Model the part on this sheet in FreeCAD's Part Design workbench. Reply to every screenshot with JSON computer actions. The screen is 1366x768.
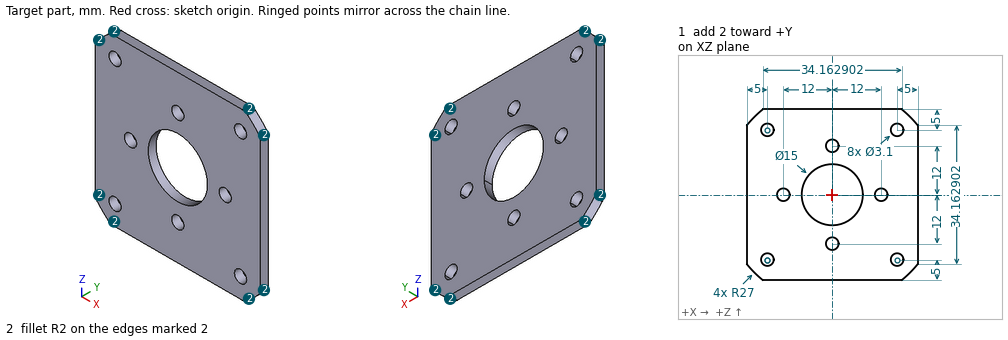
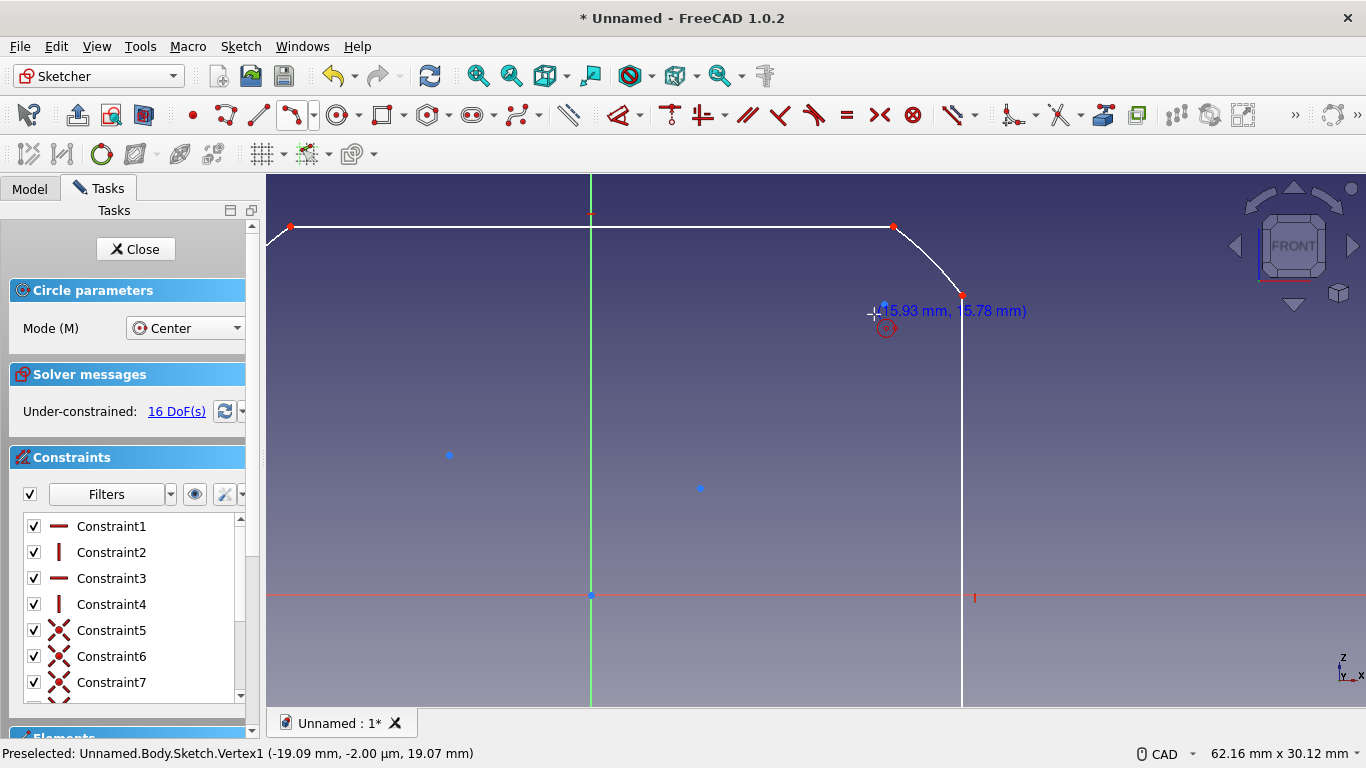
{"action": "left_click", "coordinate": [873, 314]}
{"action": "mouse_move", "coordinate": [892, 294]}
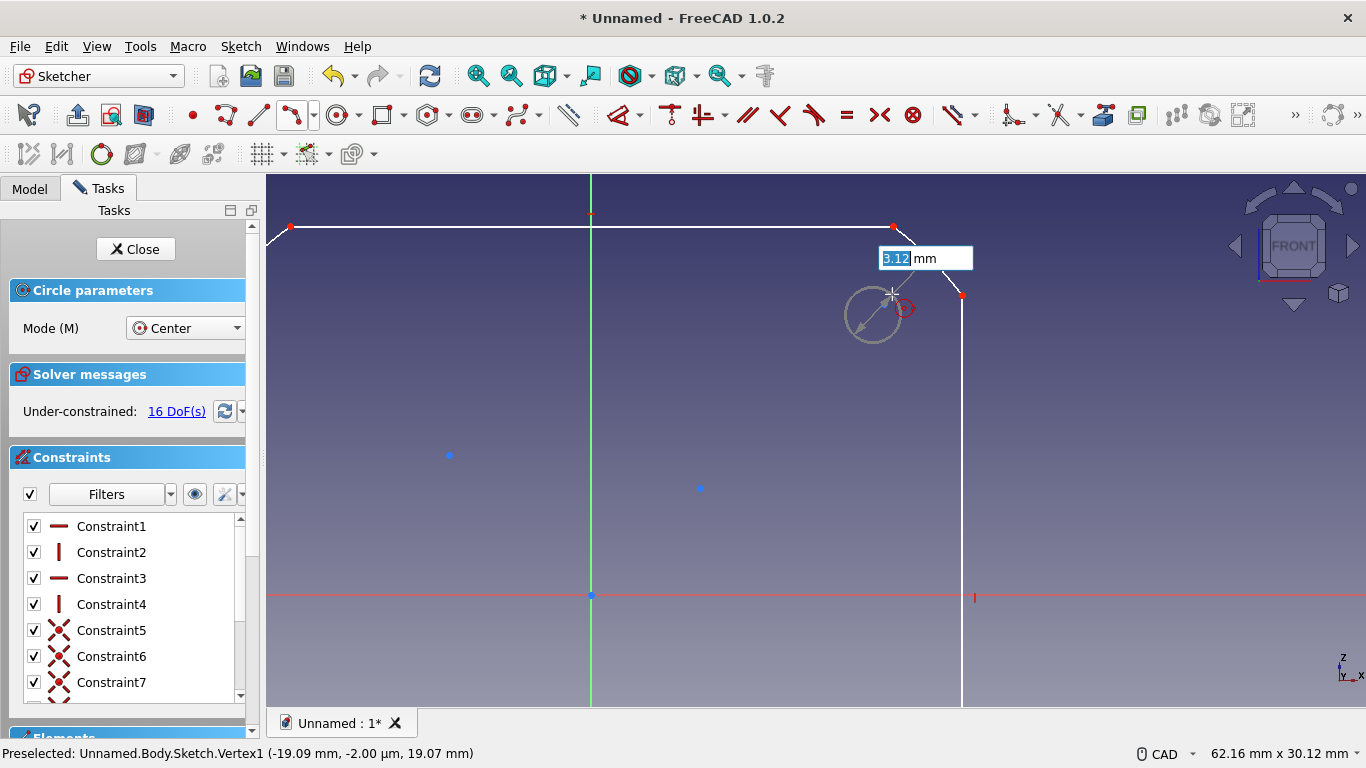
{"action": "type", "text": "3.1"}
{"action": "key", "text": "Return"}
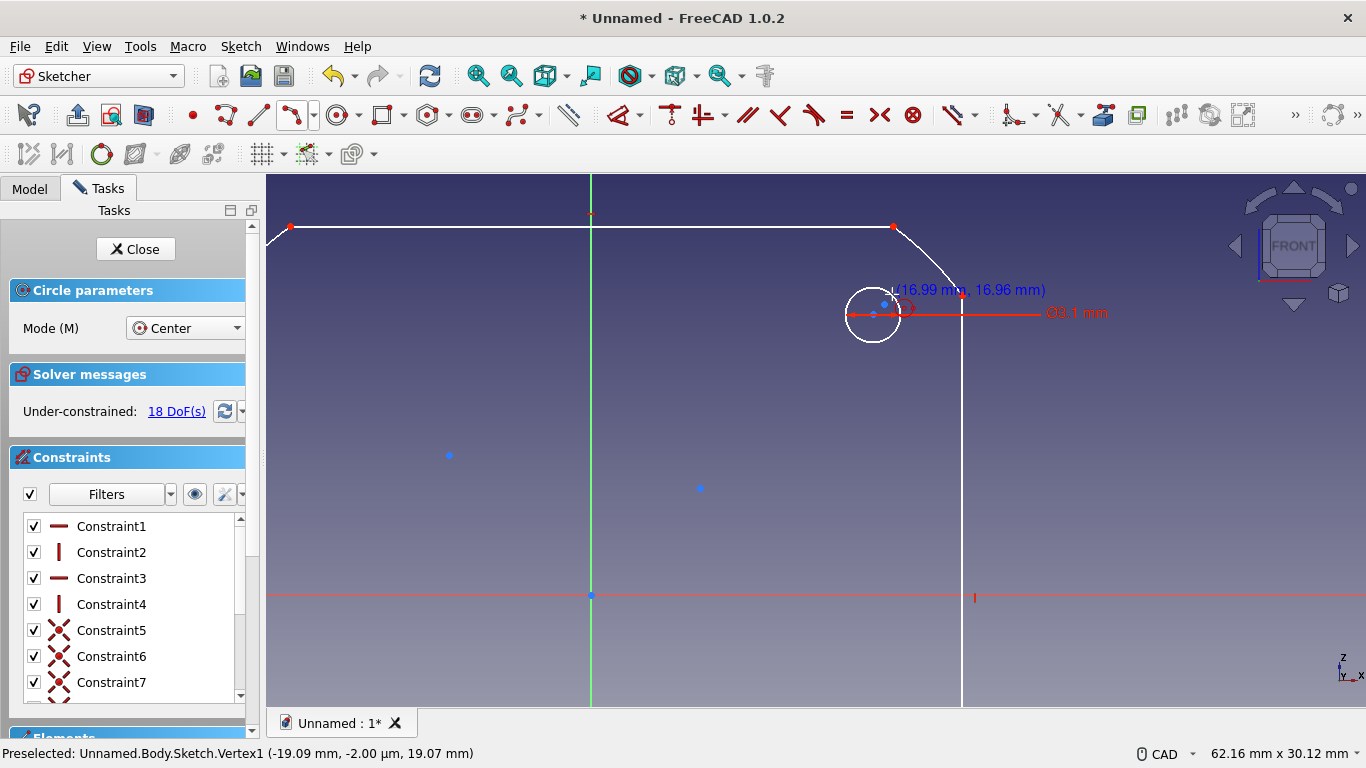
{"action": "left_click", "coordinate": [591, 383]}
{"action": "mouse_move", "coordinate": [611, 363]}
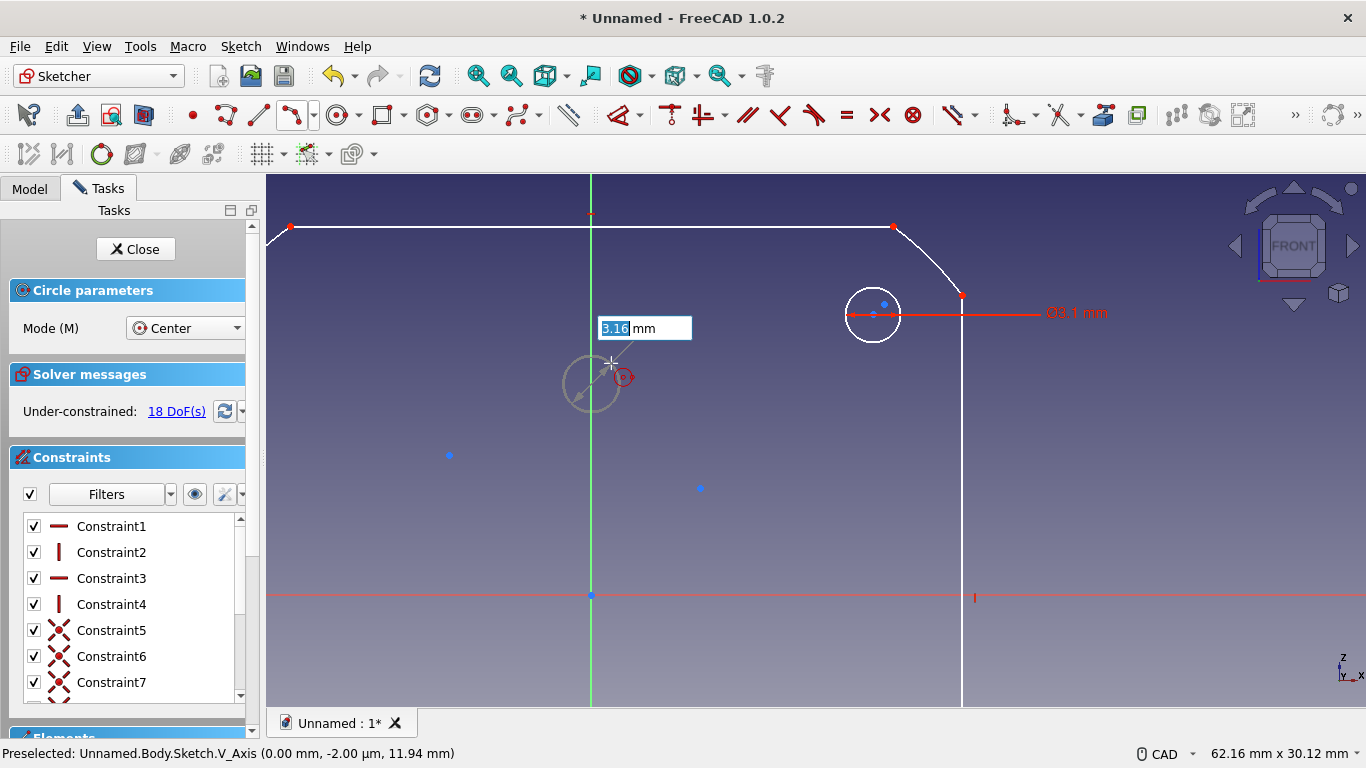
{"action": "type", "text": "3.1"}
{"action": "key", "text": "Return"}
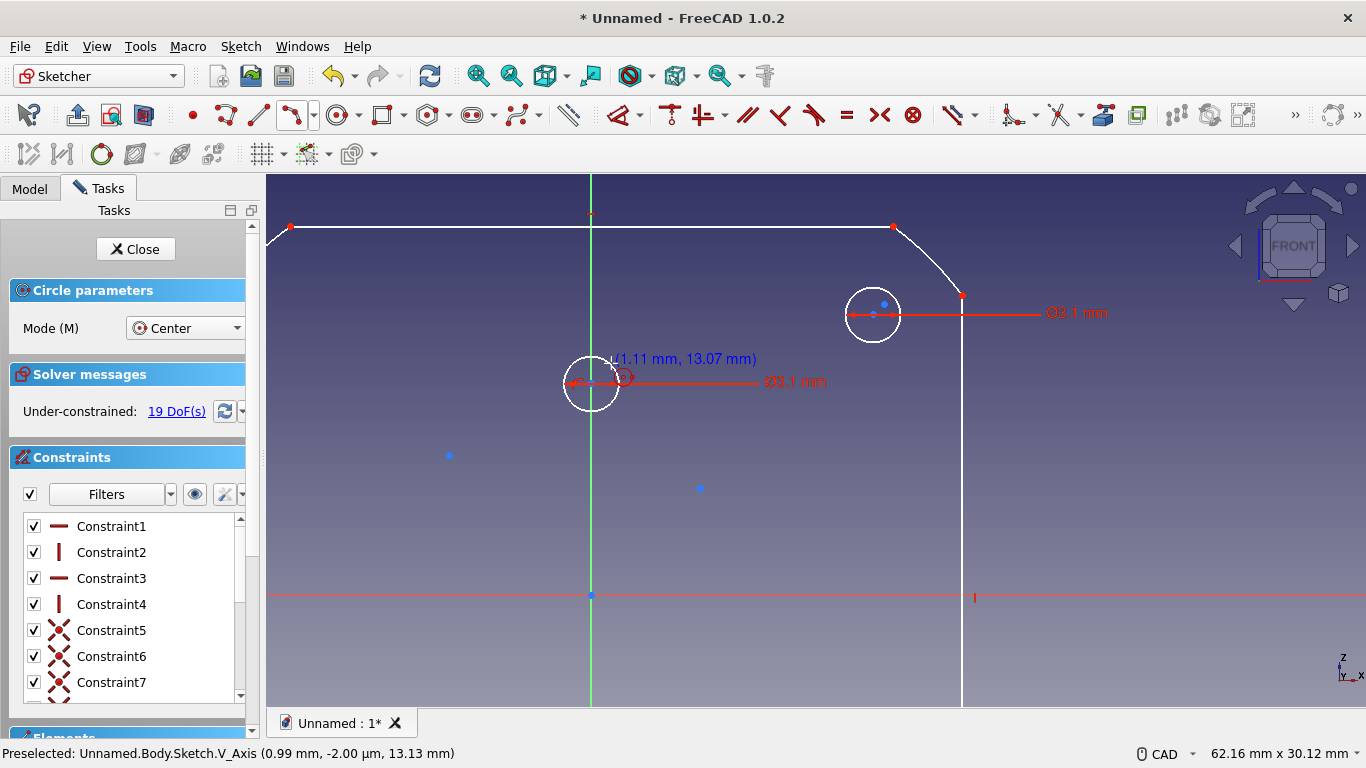
{"action": "left_click", "coordinate": [310, 314]}
{"action": "mouse_move", "coordinate": [329, 294]}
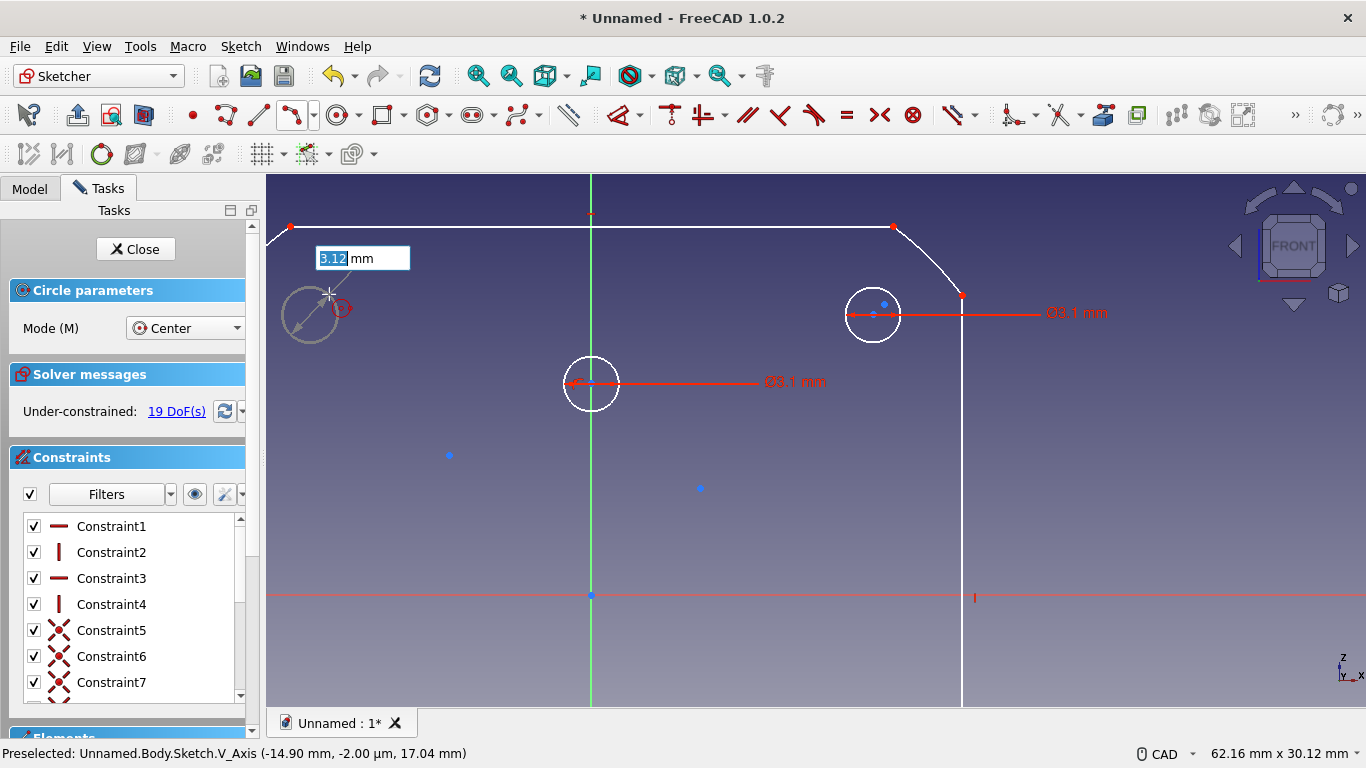
{"action": "type", "text": "3.1"}
{"action": "key", "text": "Return"}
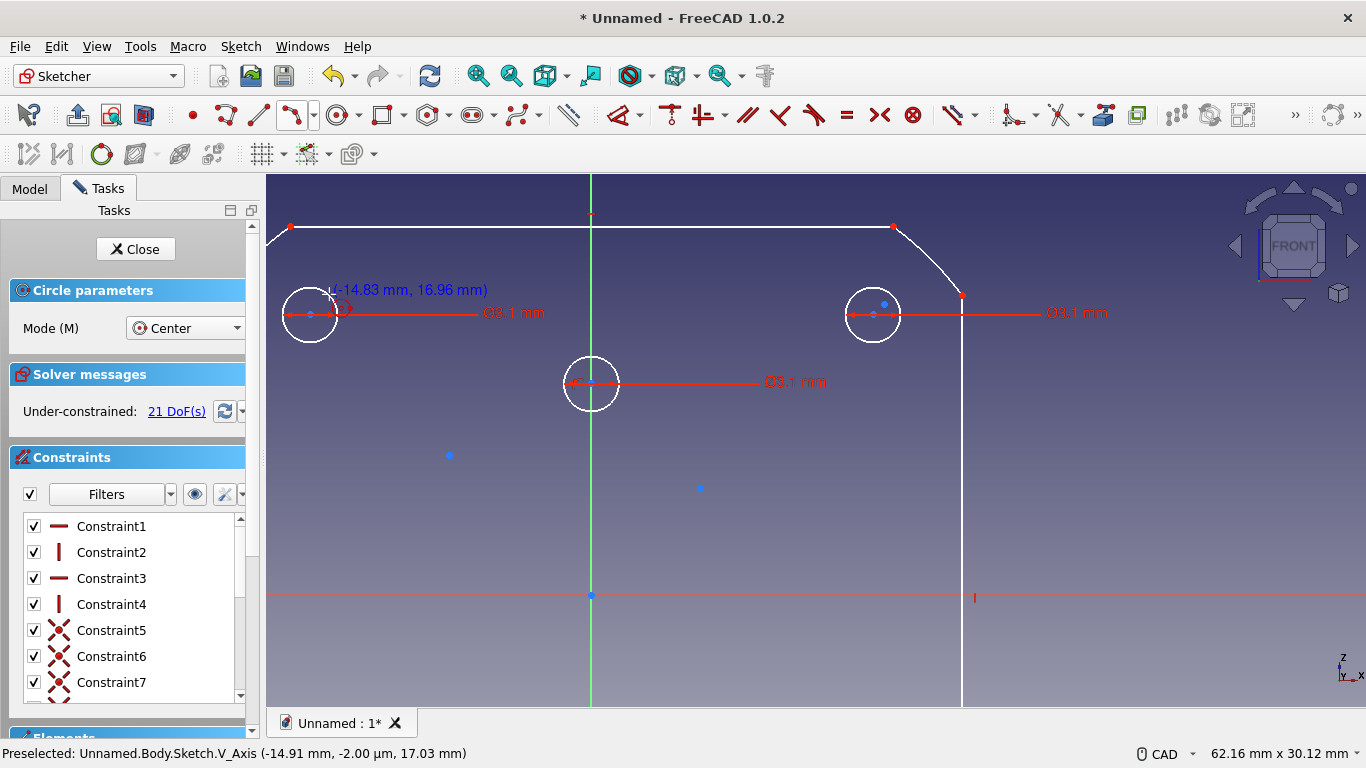
{"action": "left_click", "coordinate": [804, 595]}
{"action": "mouse_move", "coordinate": [823, 576]}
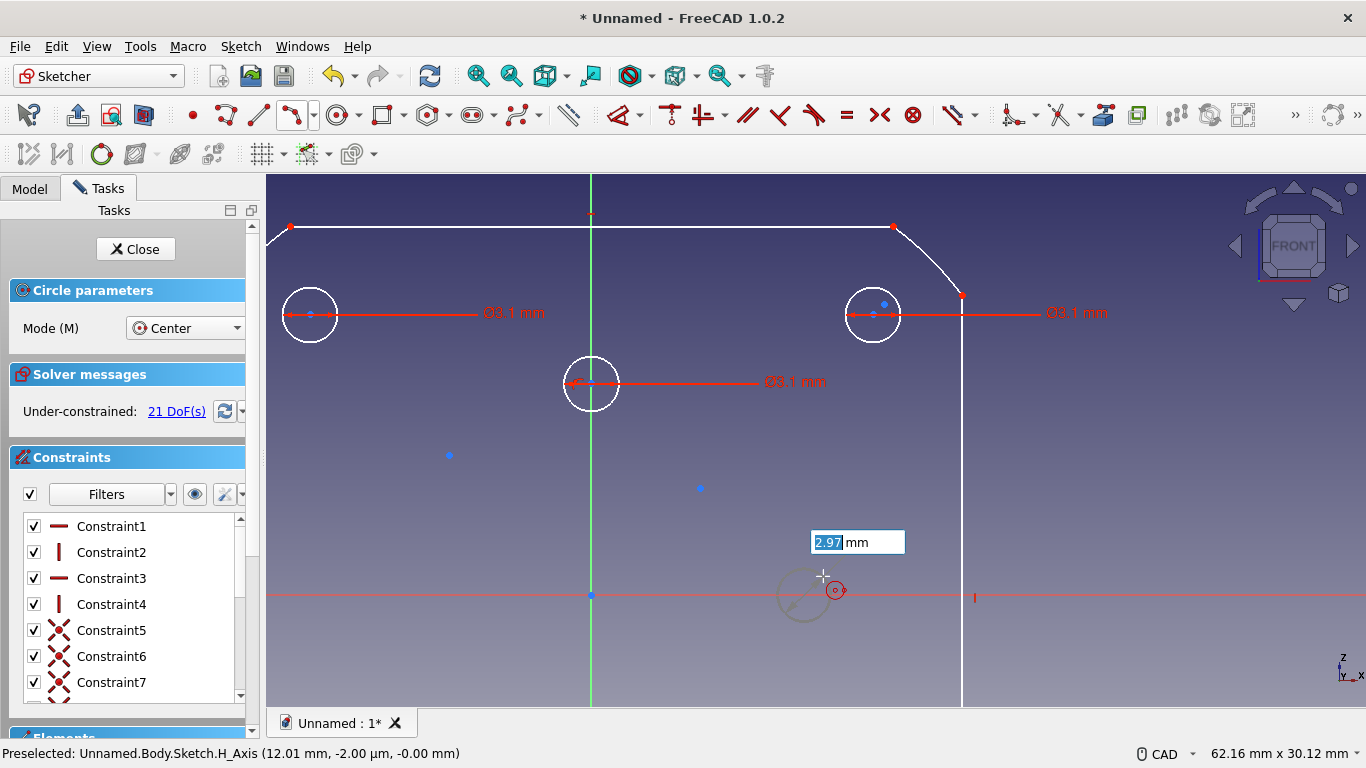
{"action": "type", "text": "3.1"}
{"action": "key", "text": "Return"}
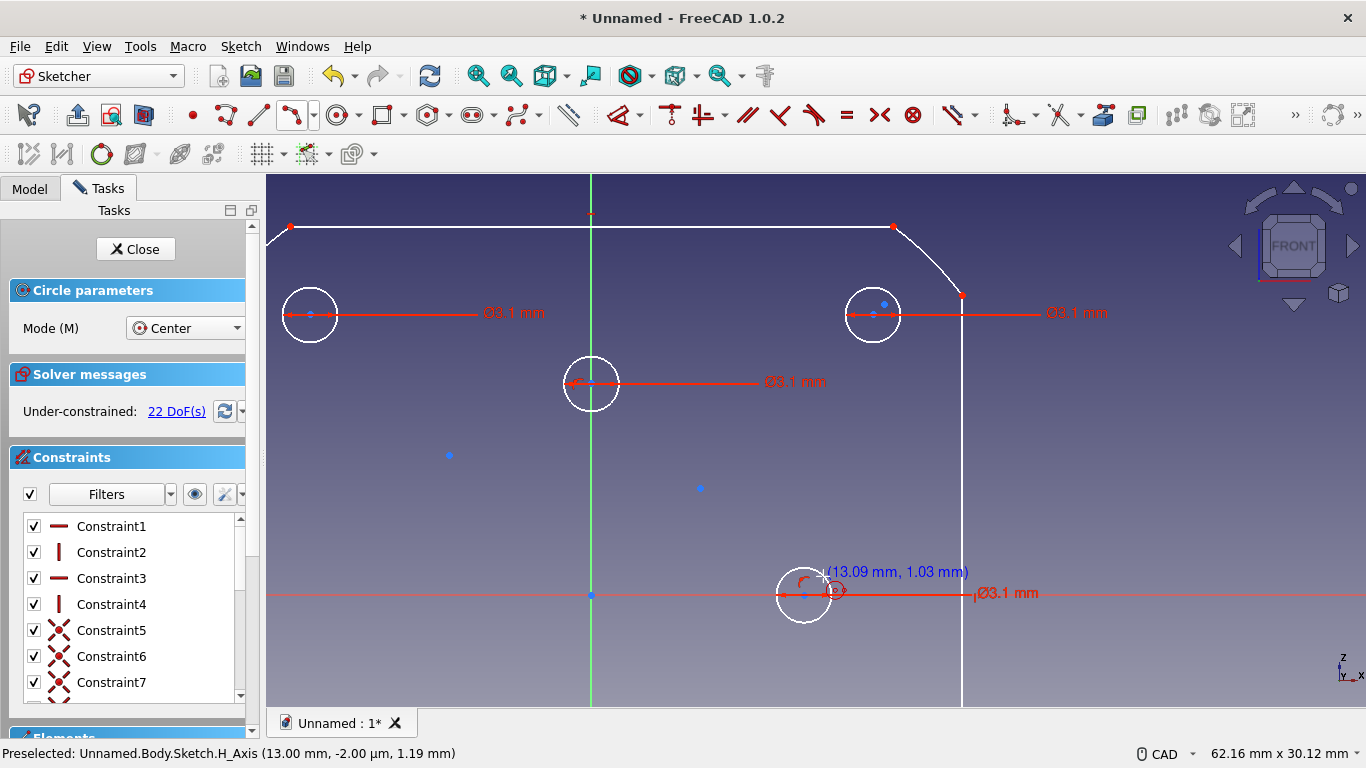
{"action": "scroll", "coordinate": [875, 314], "scroll_direction": "down", "scroll_amount": 4}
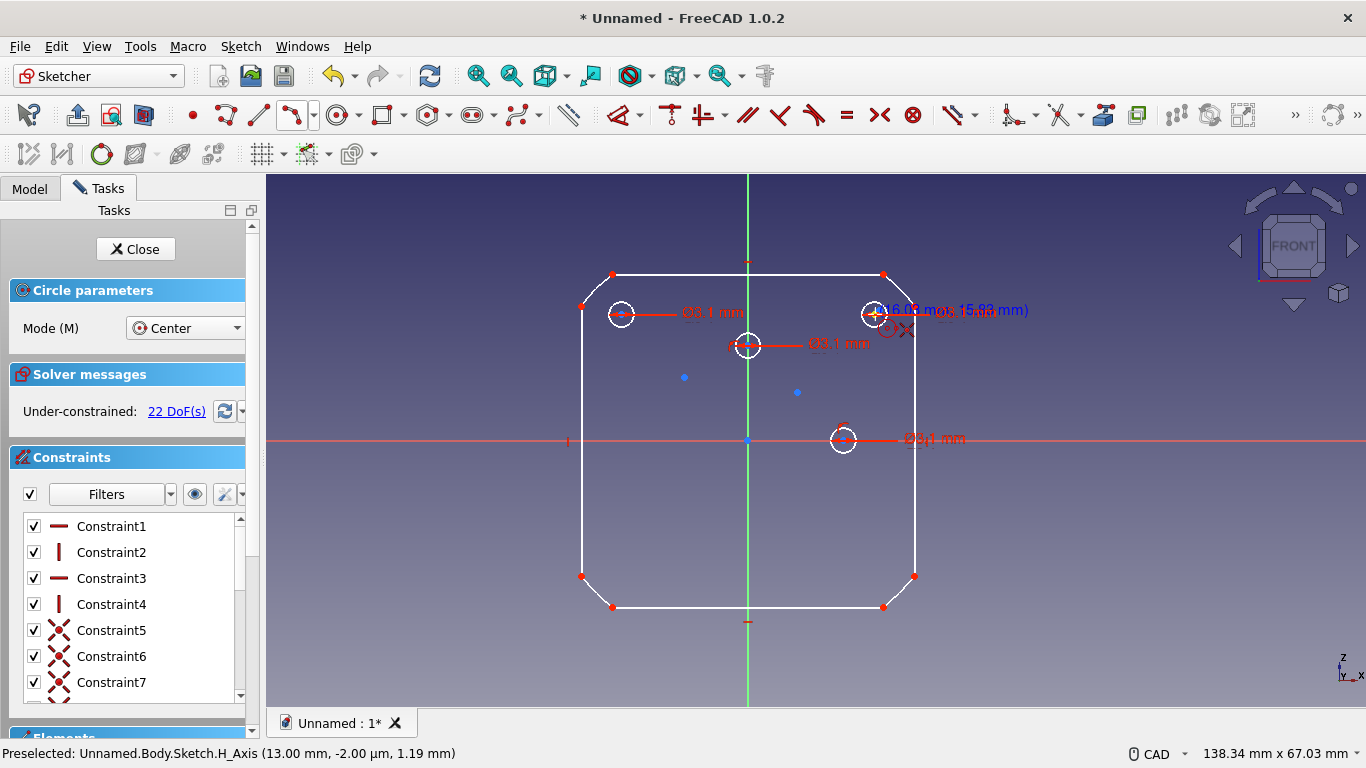
{"action": "scroll", "coordinate": [874, 567], "scroll_direction": "up", "scroll_amount": 4}